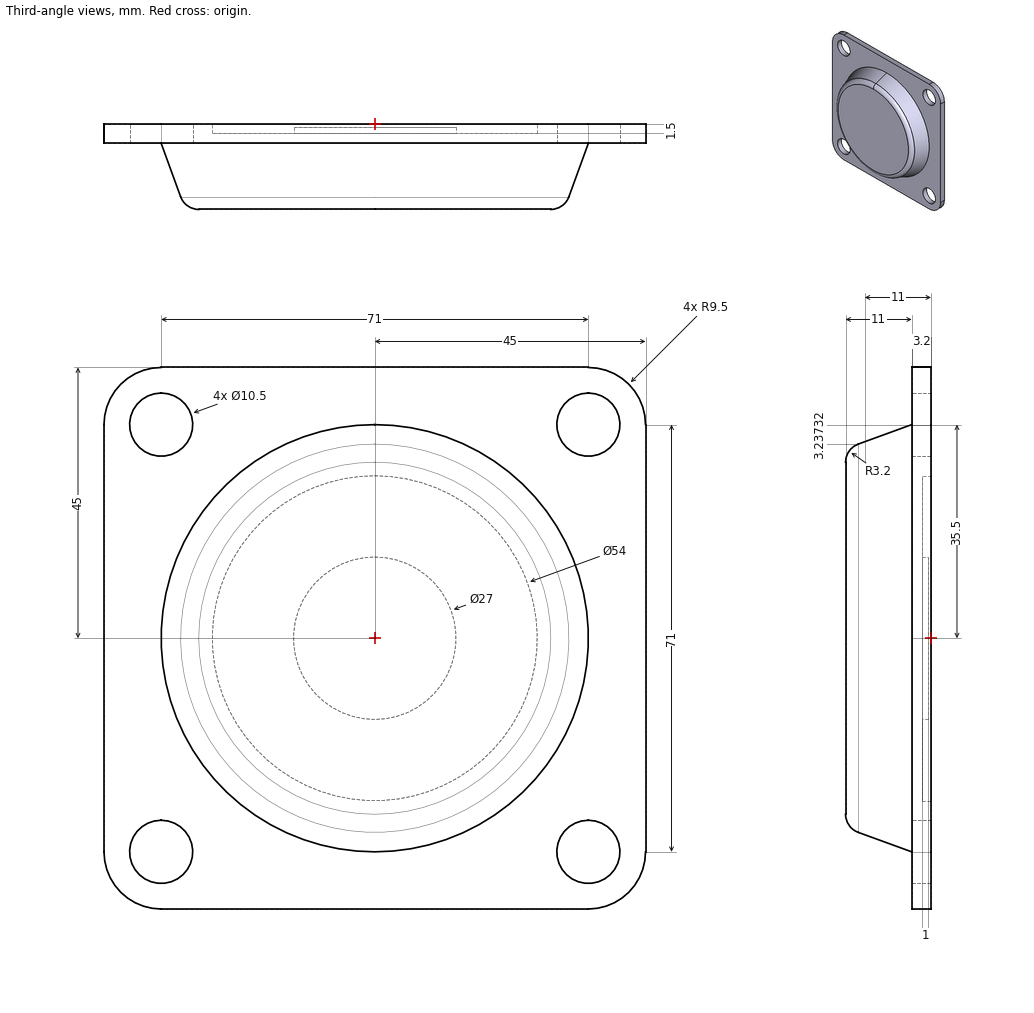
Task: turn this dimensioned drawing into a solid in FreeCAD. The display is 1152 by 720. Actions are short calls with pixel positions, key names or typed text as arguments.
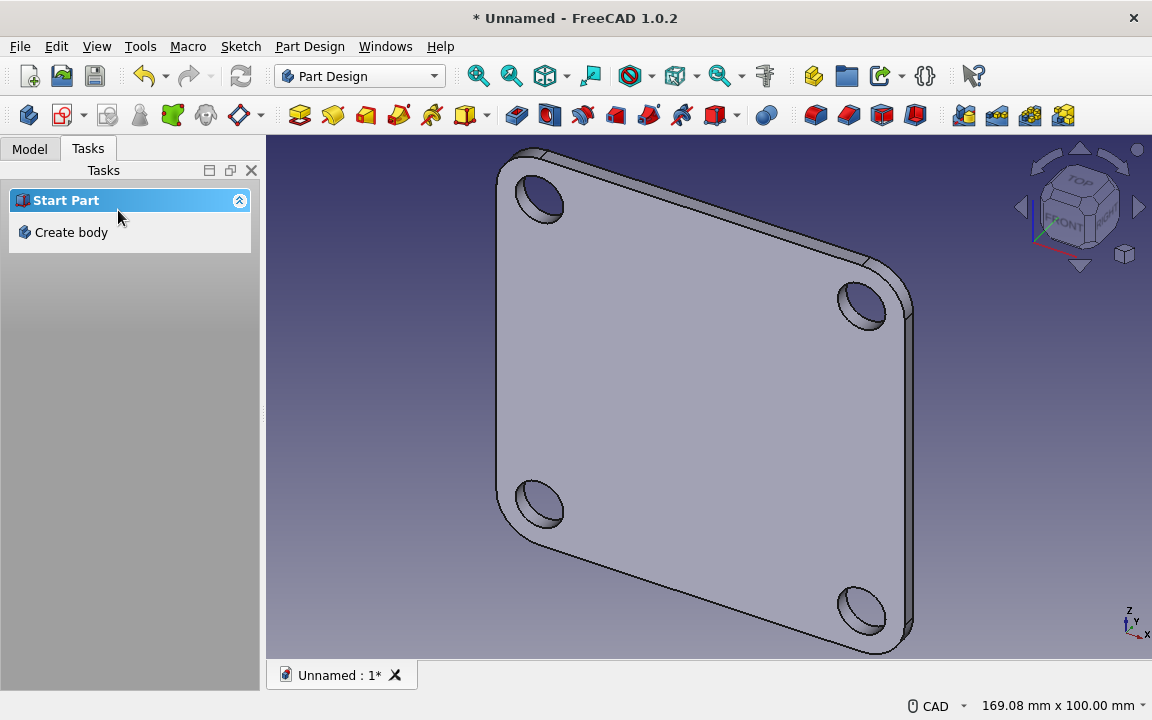
key(v)
key(f)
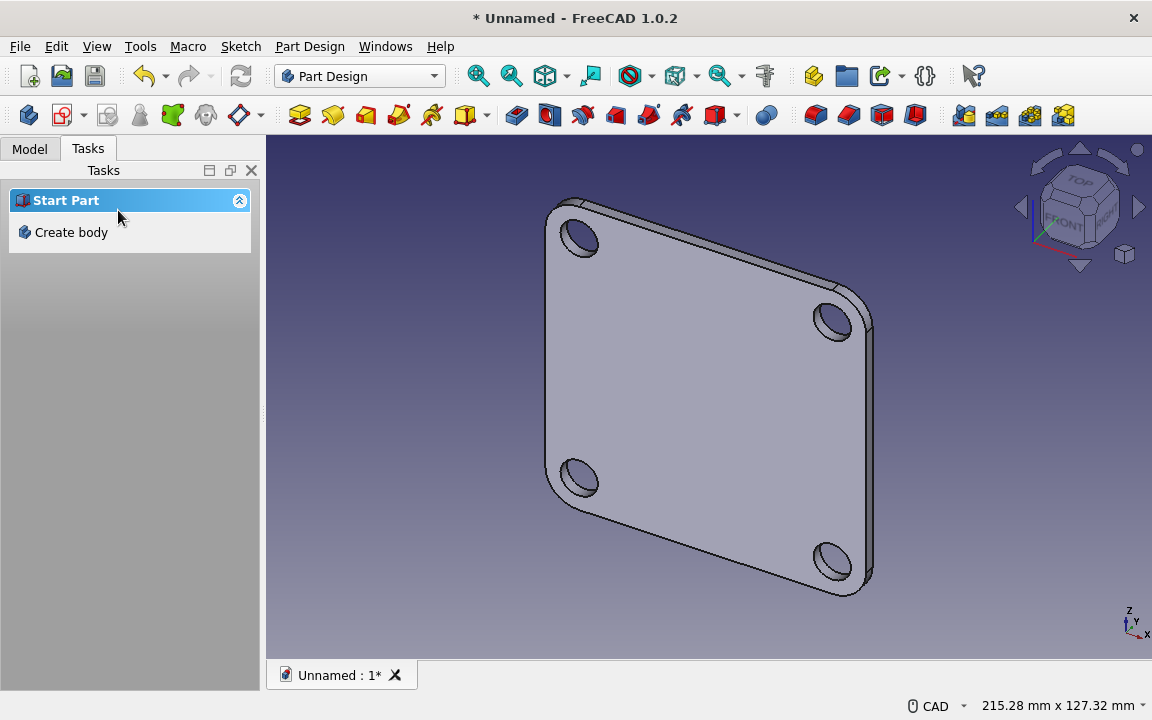
key(4)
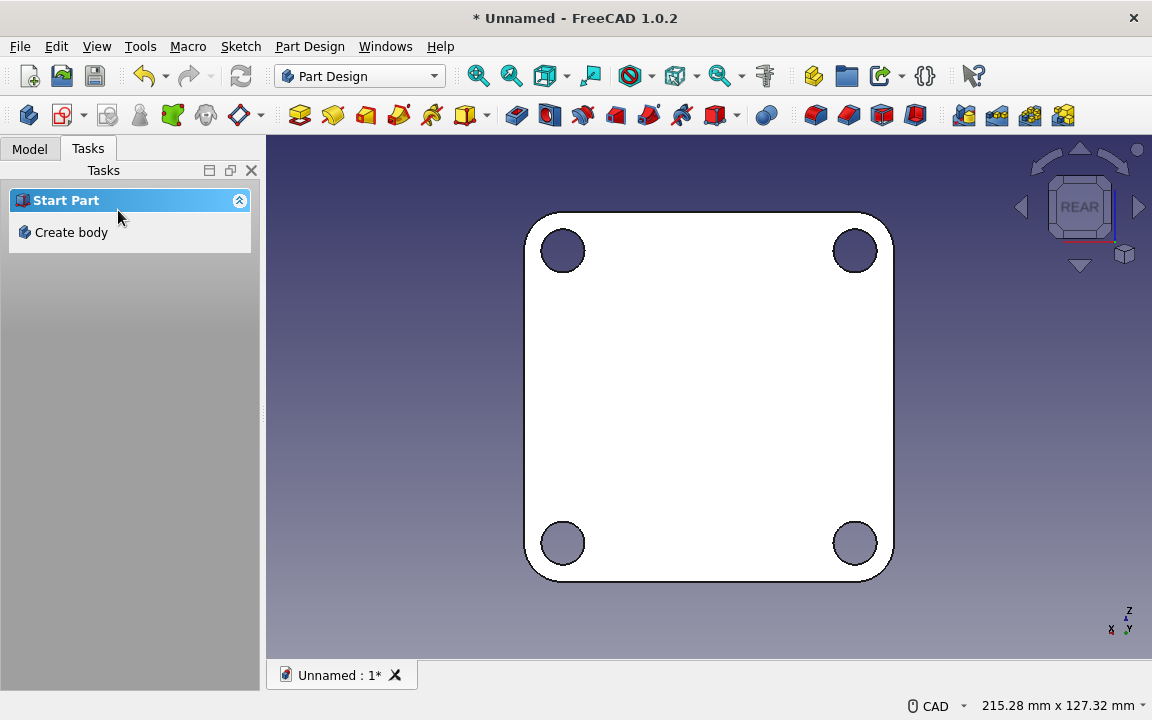
click(709, 396)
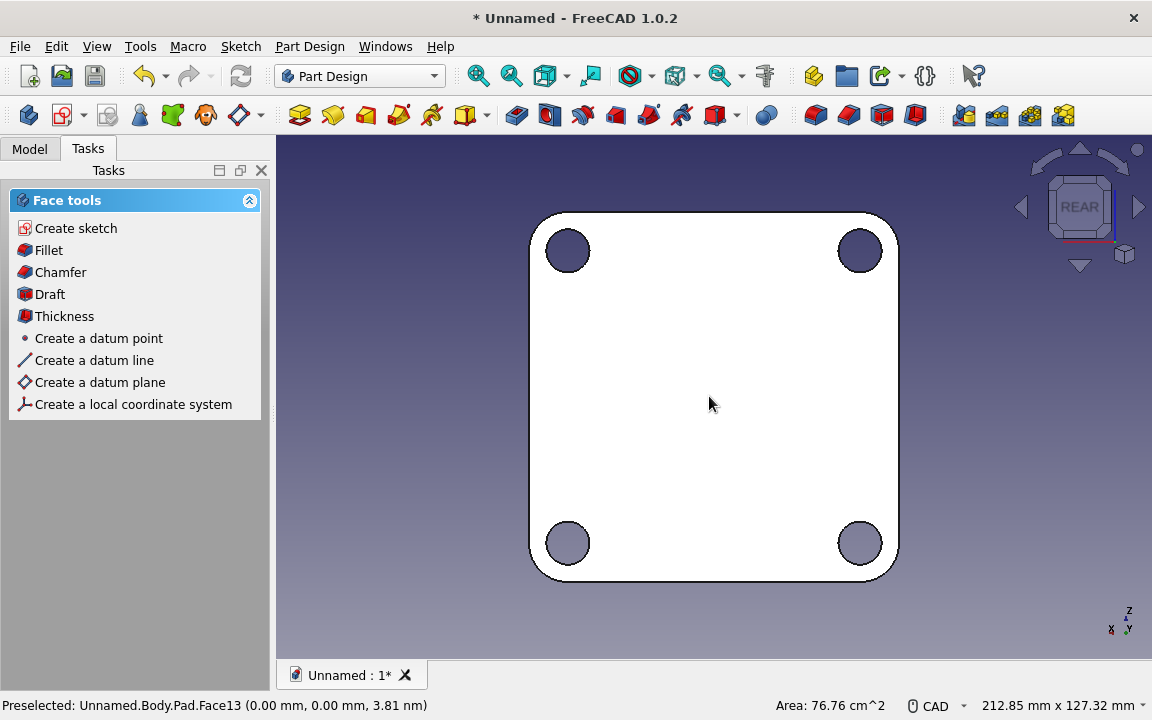
click(62, 116)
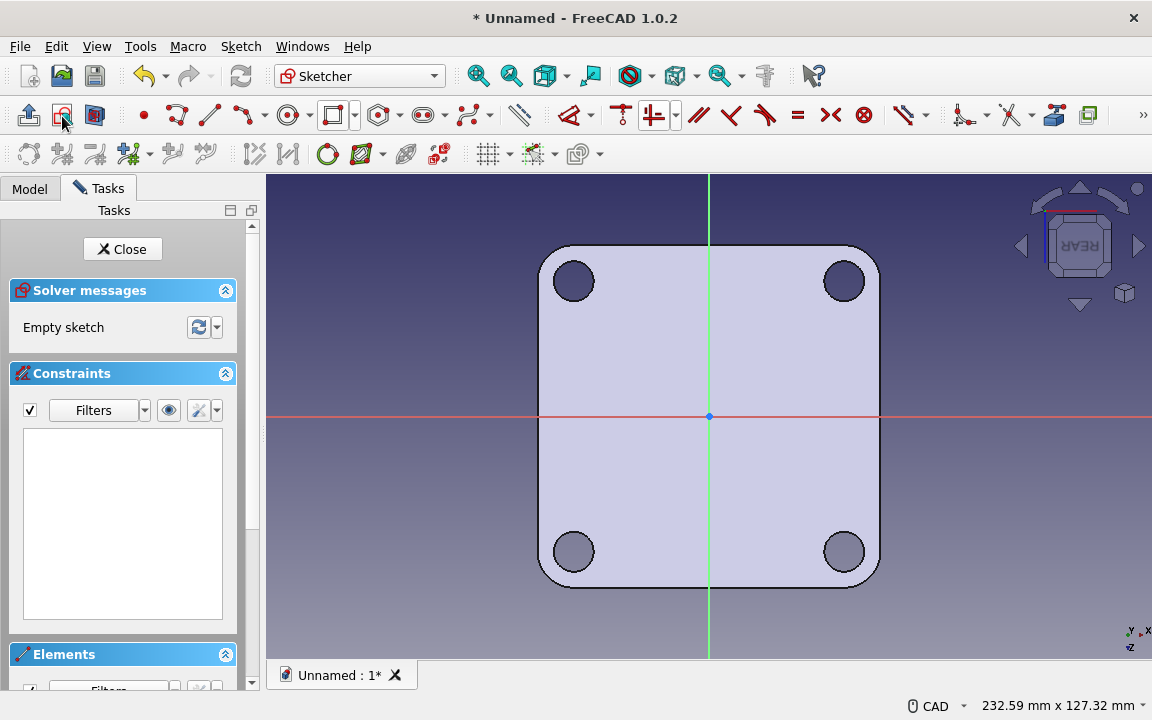
scroll(848, 416, up, 2)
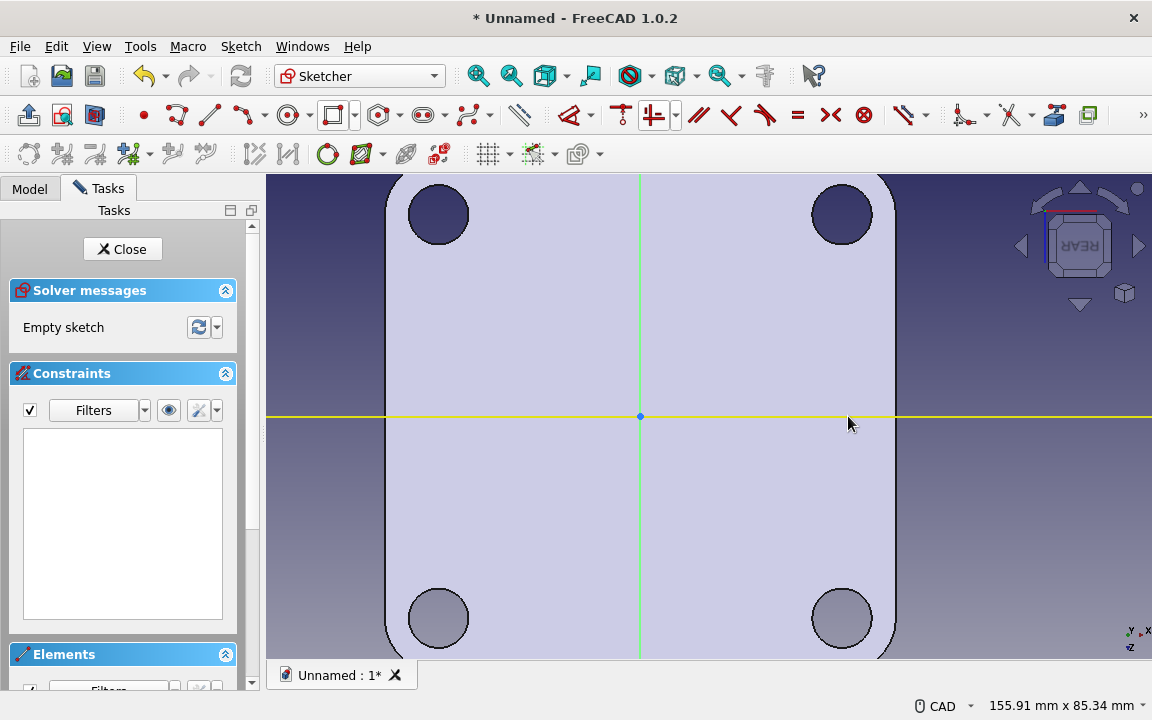
key(g)
key(c)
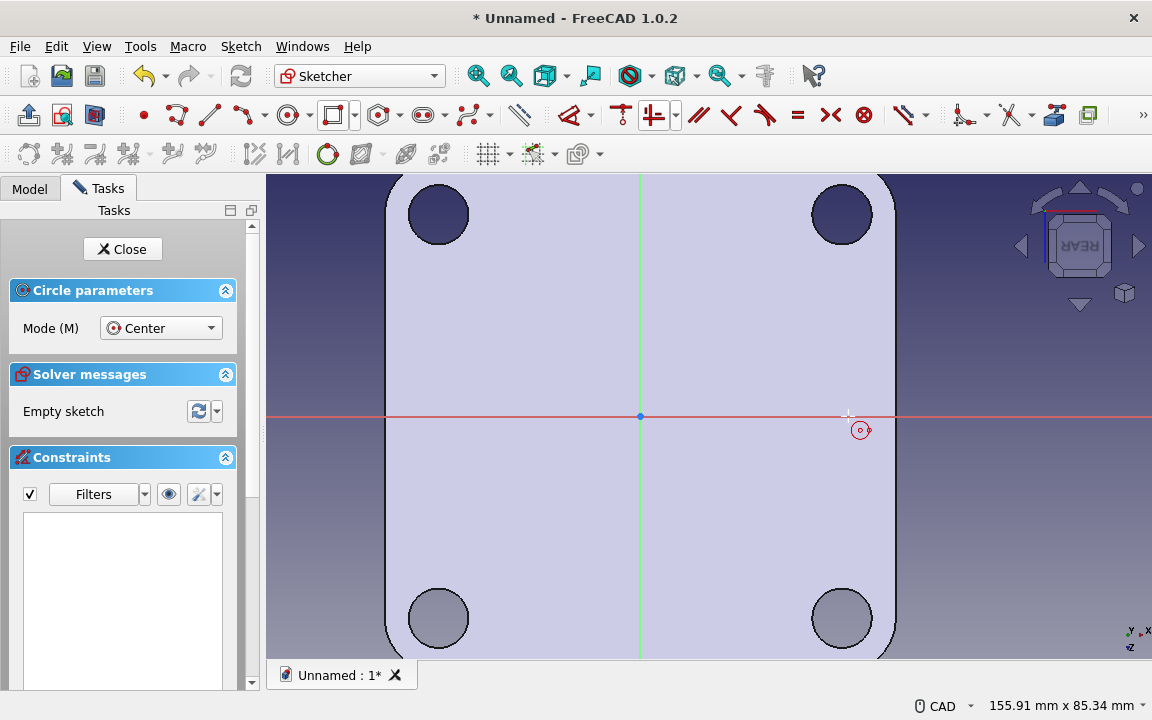
click(640, 416)
move(749, 308)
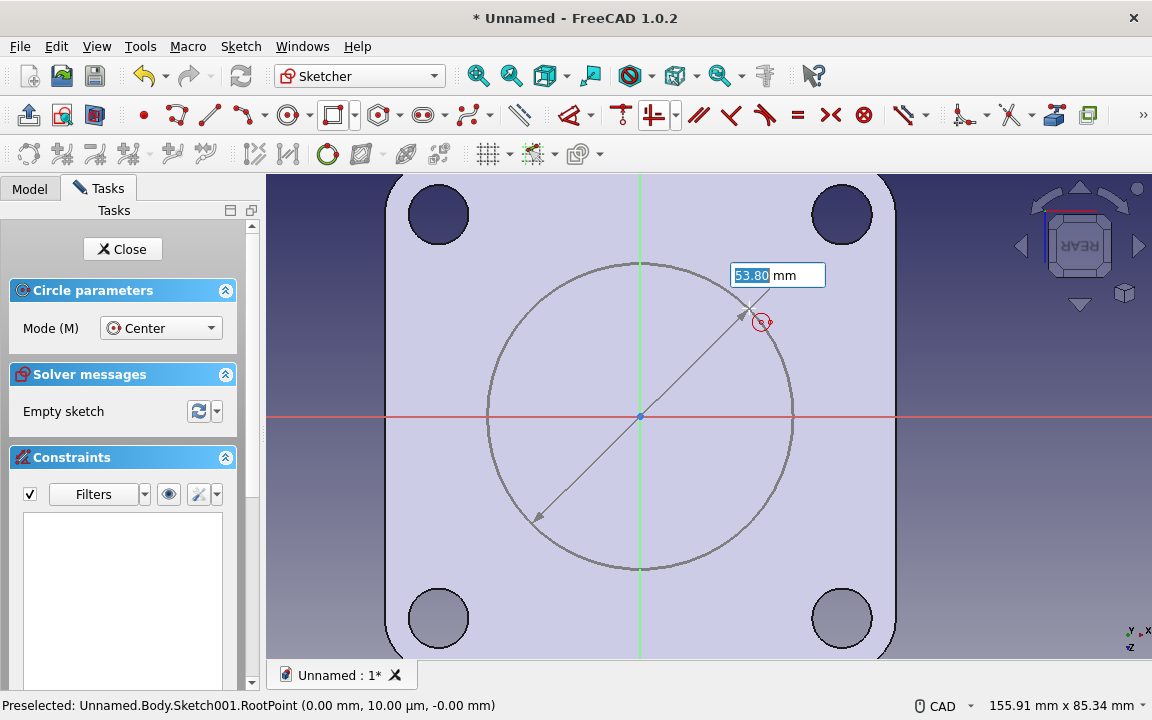
text(54)
key(Return)
key(Escape)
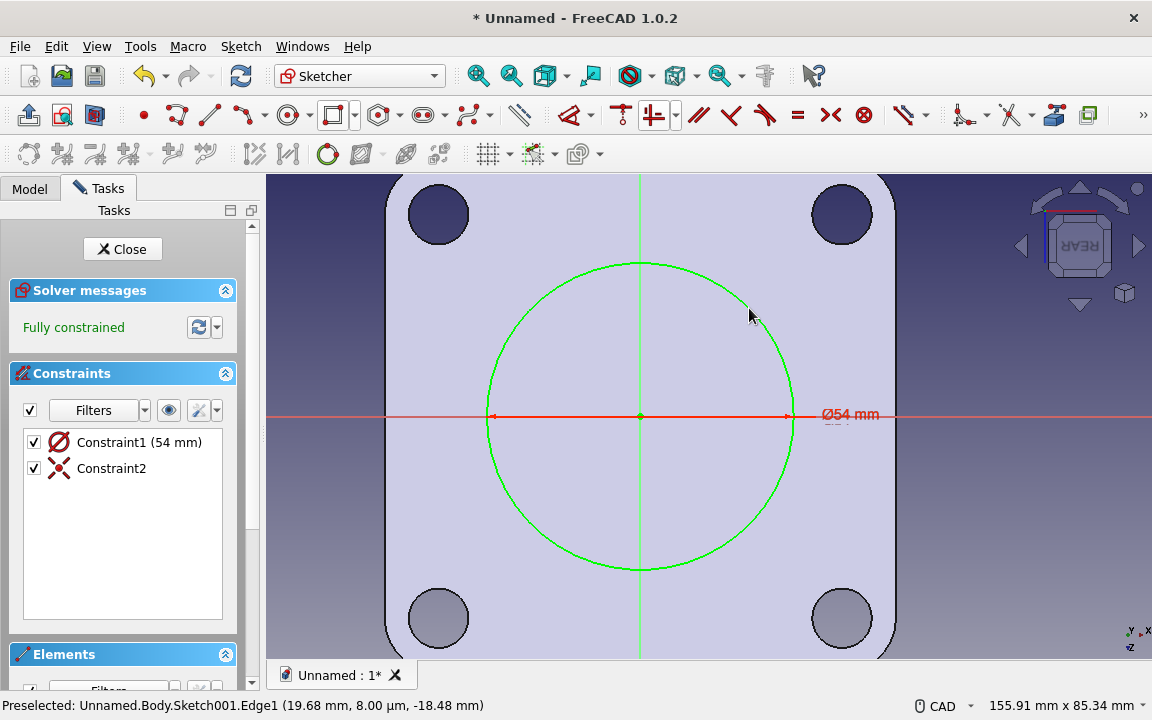
click(123, 249)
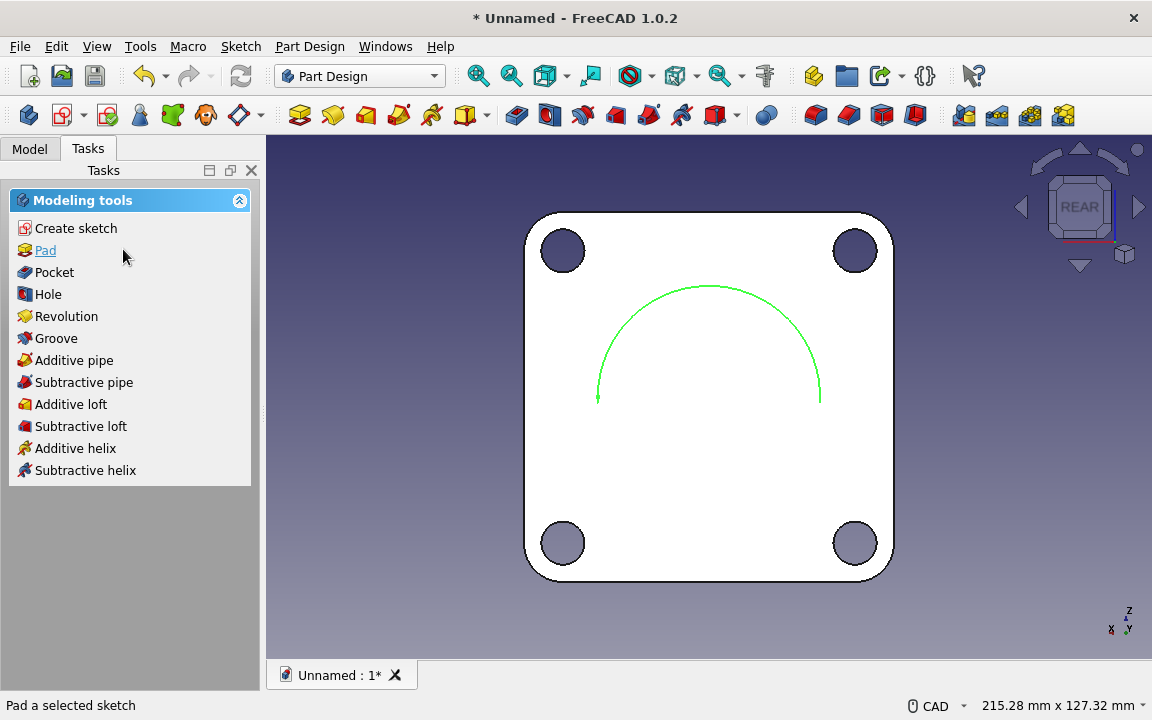
click(517, 116)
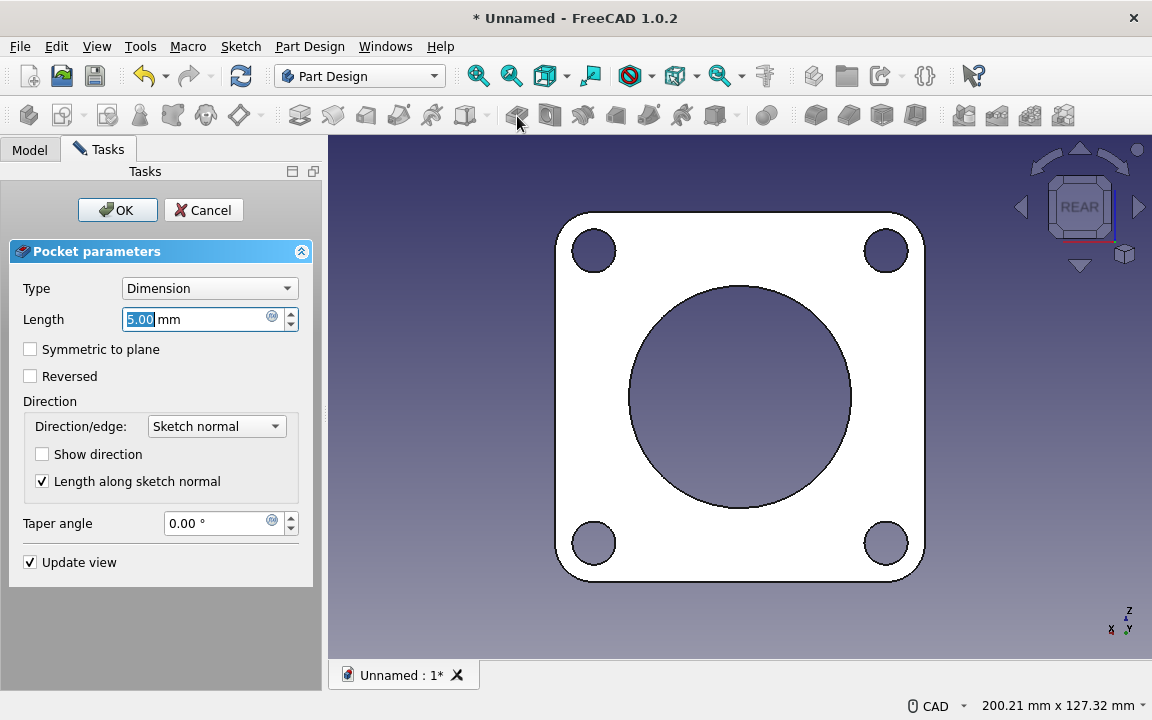
text(1.5)
key(Tab)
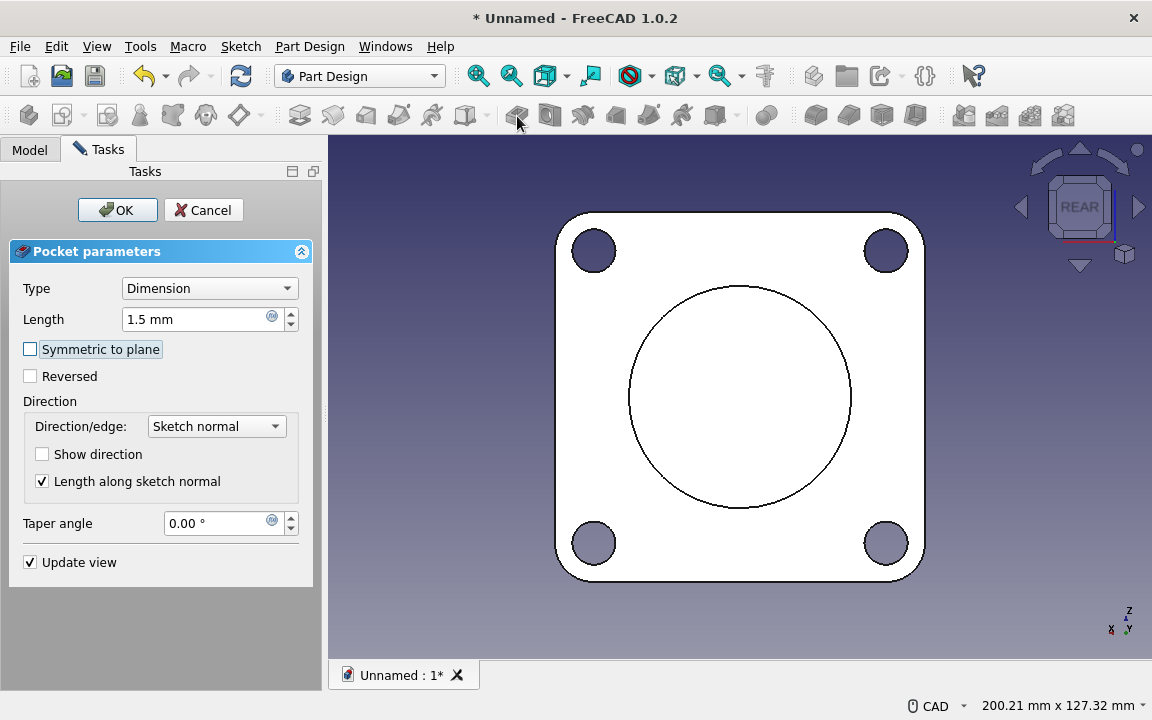
click(118, 210)